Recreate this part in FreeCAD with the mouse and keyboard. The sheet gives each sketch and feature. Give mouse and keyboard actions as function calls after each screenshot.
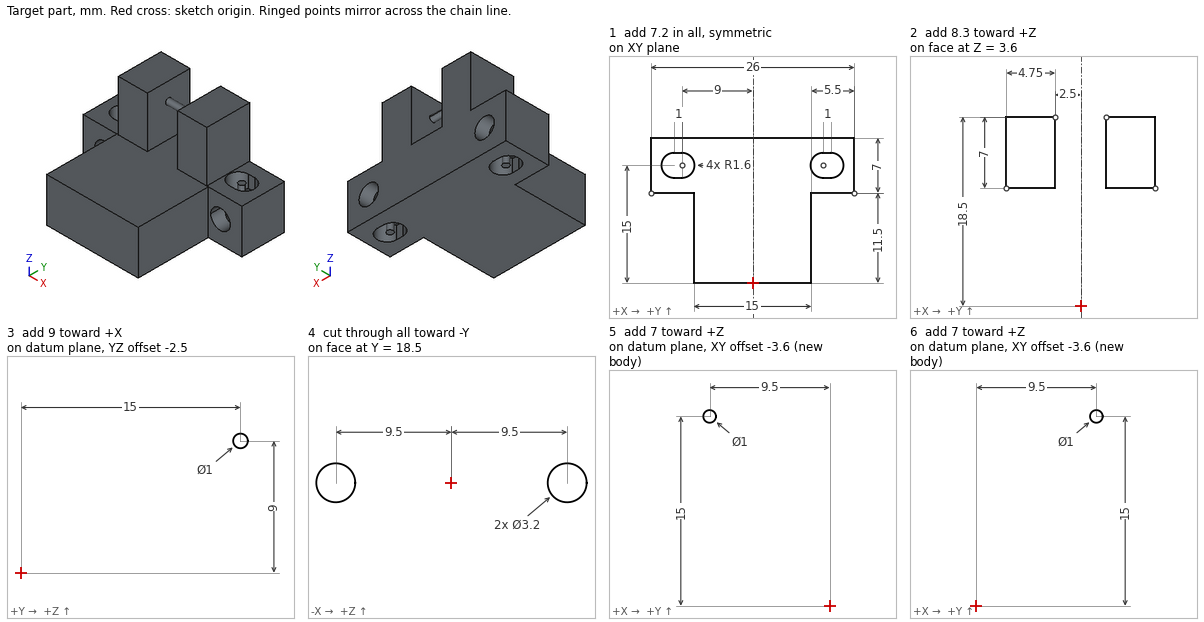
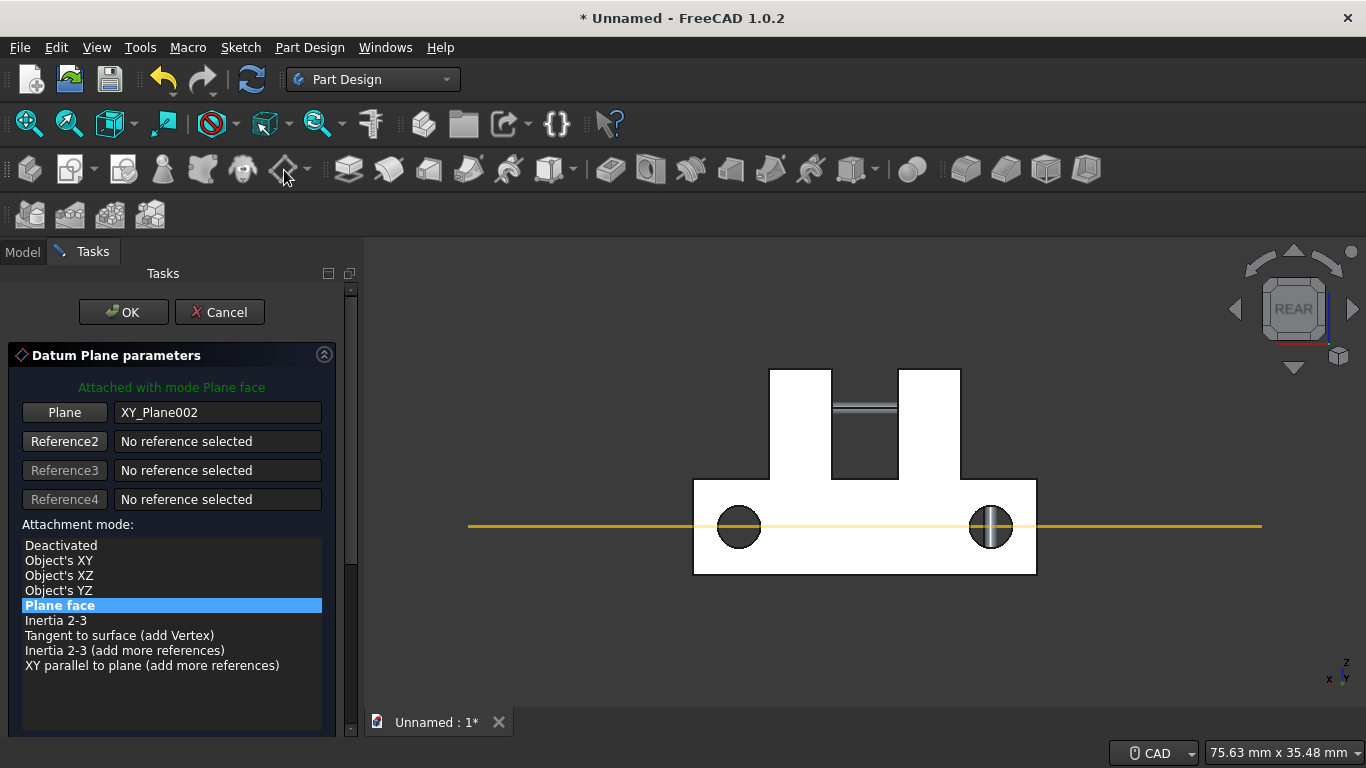
scroll(351, 510, down, 3)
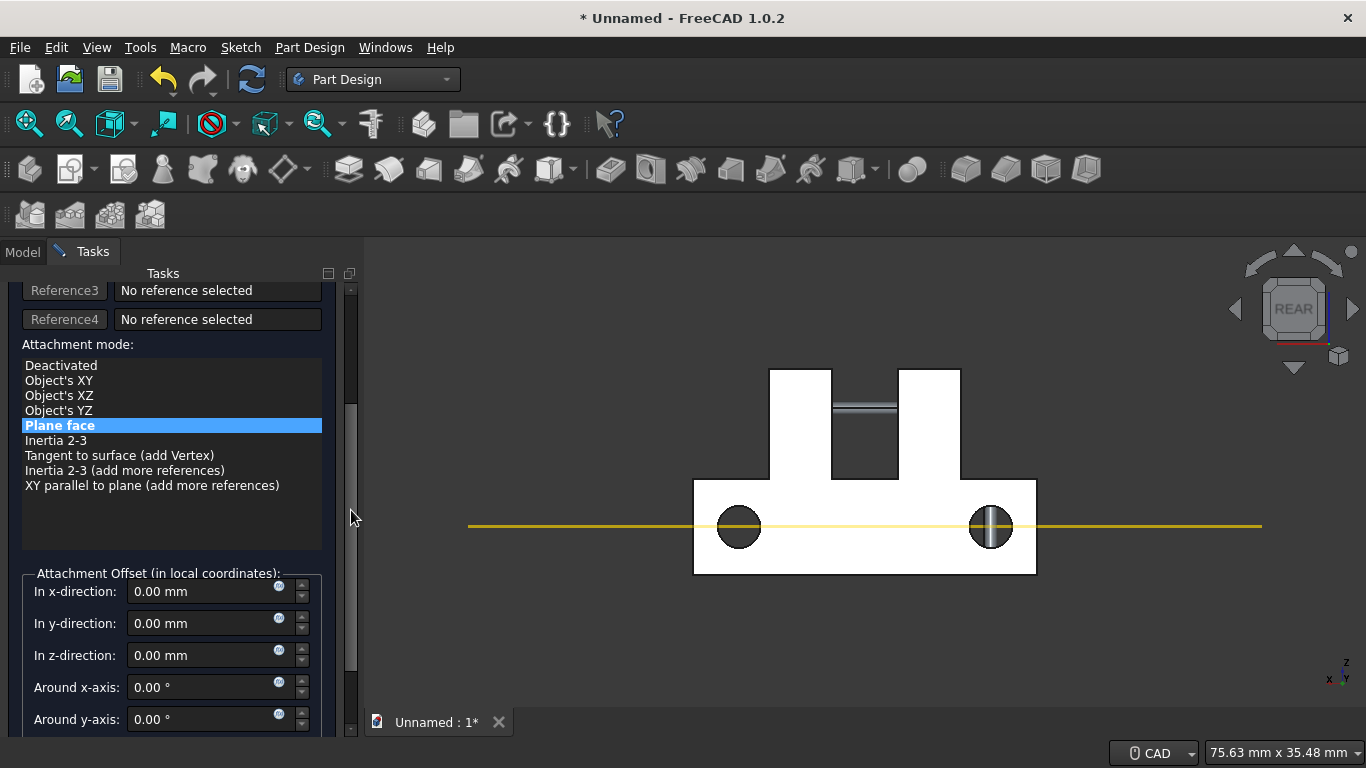
triple_click(210, 655)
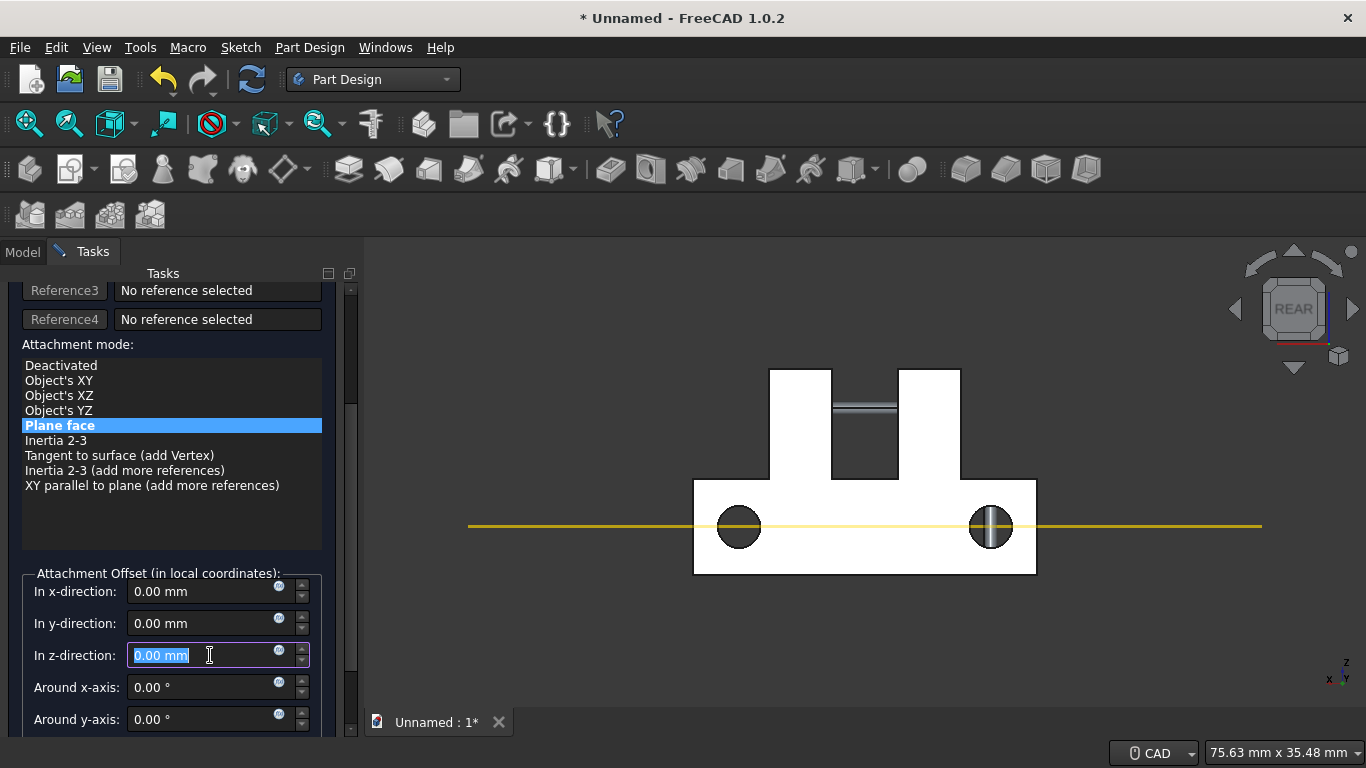
text(-3.6)
key(Tab)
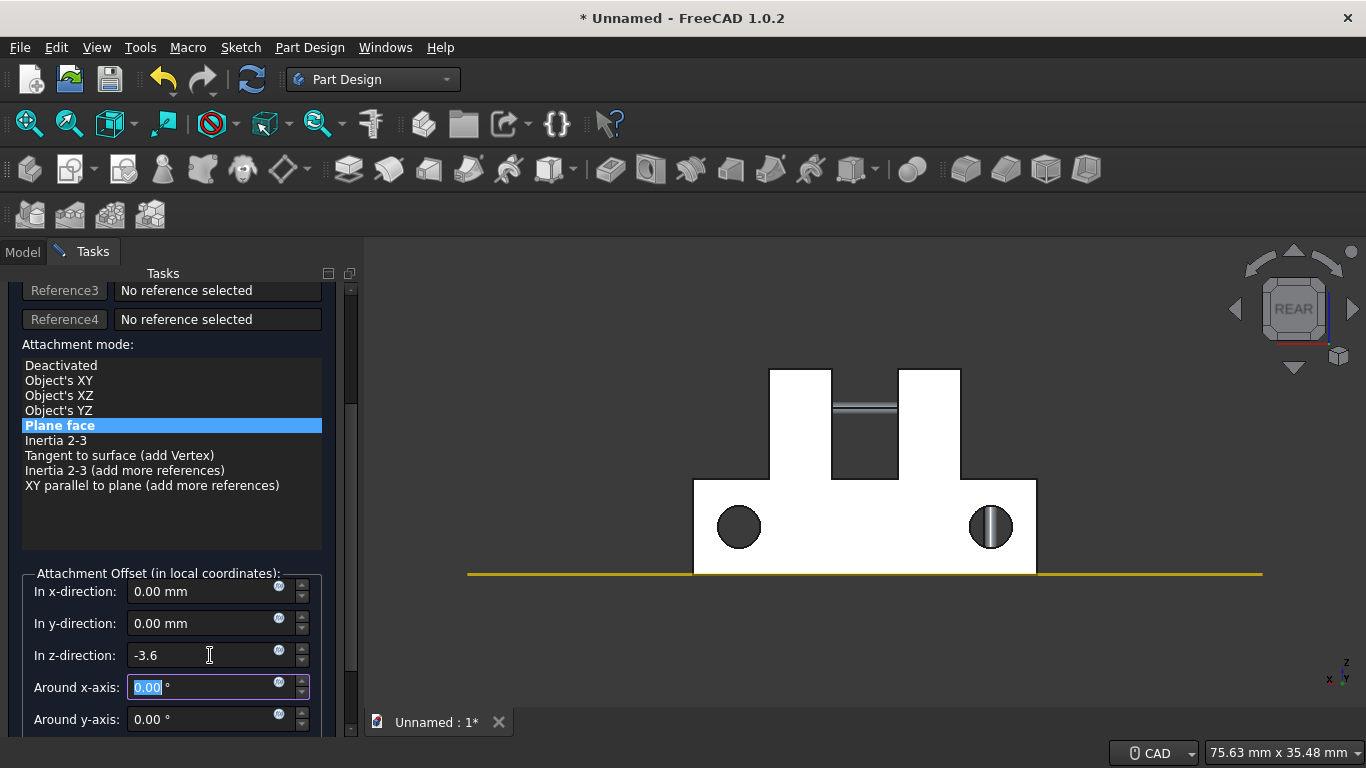
scroll(351, 510, up, 4)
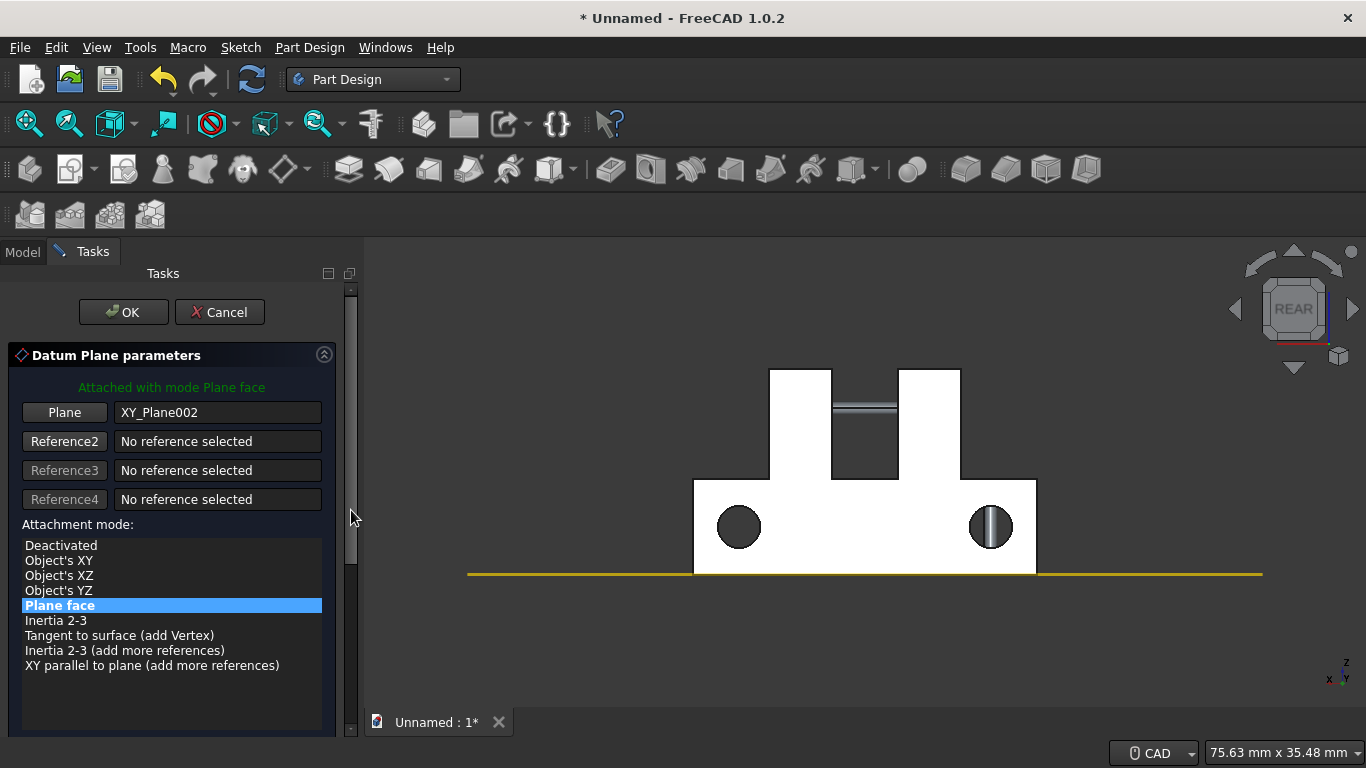
click(124, 312)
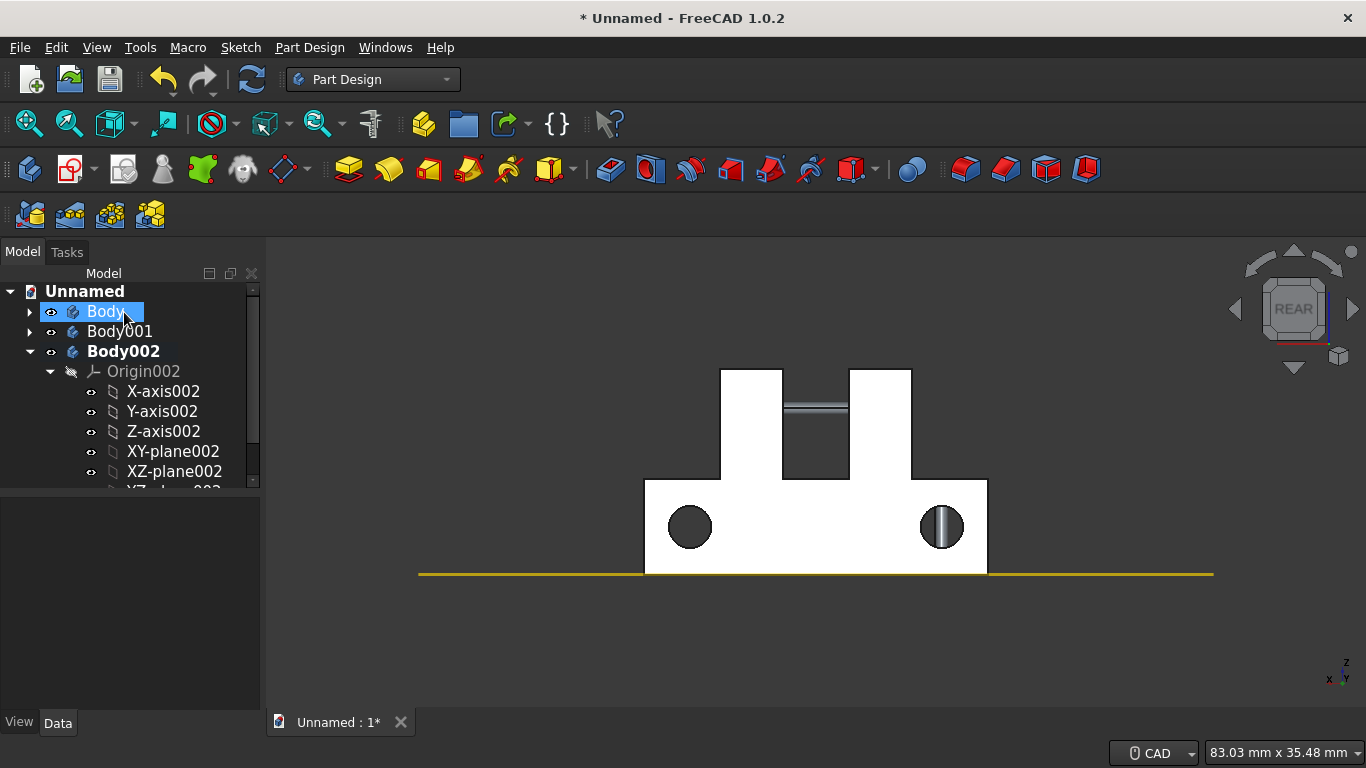
scroll(100, 387, down, 3)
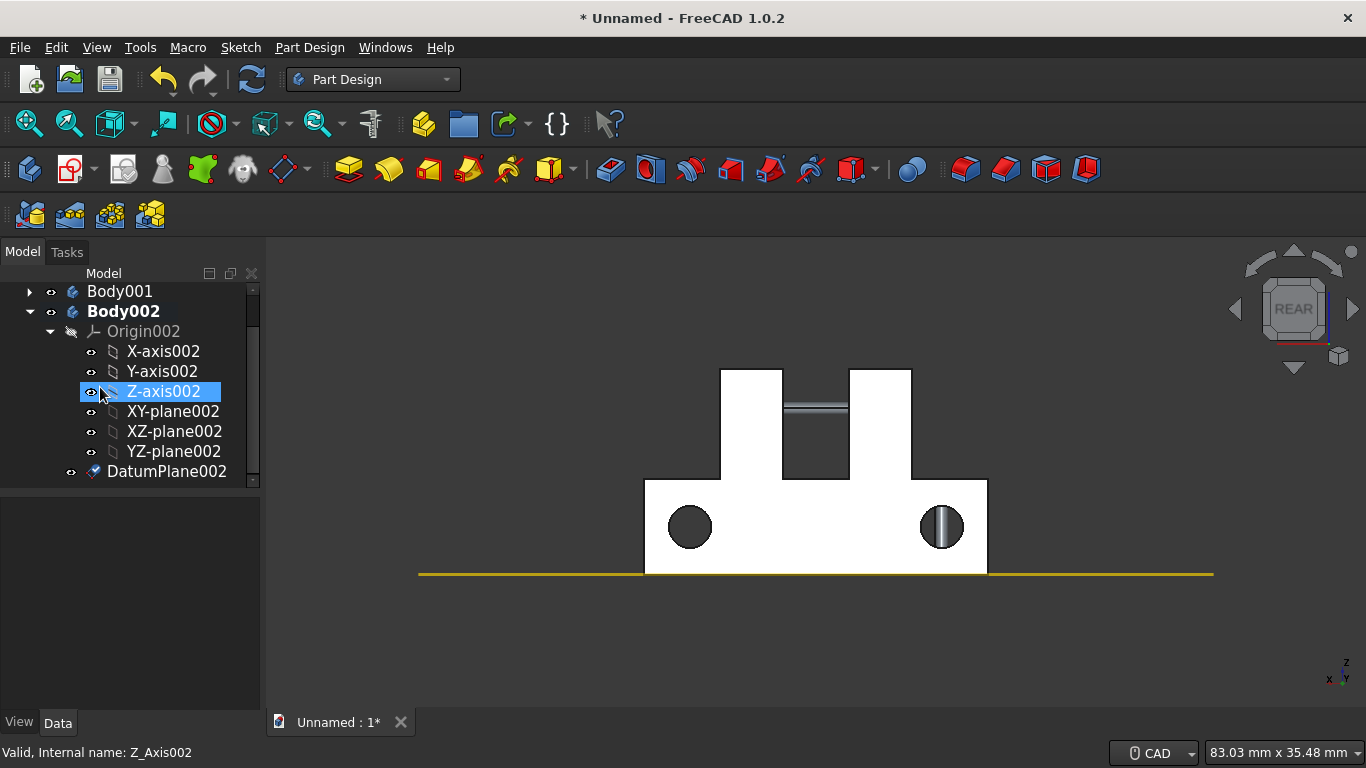
click(116, 472)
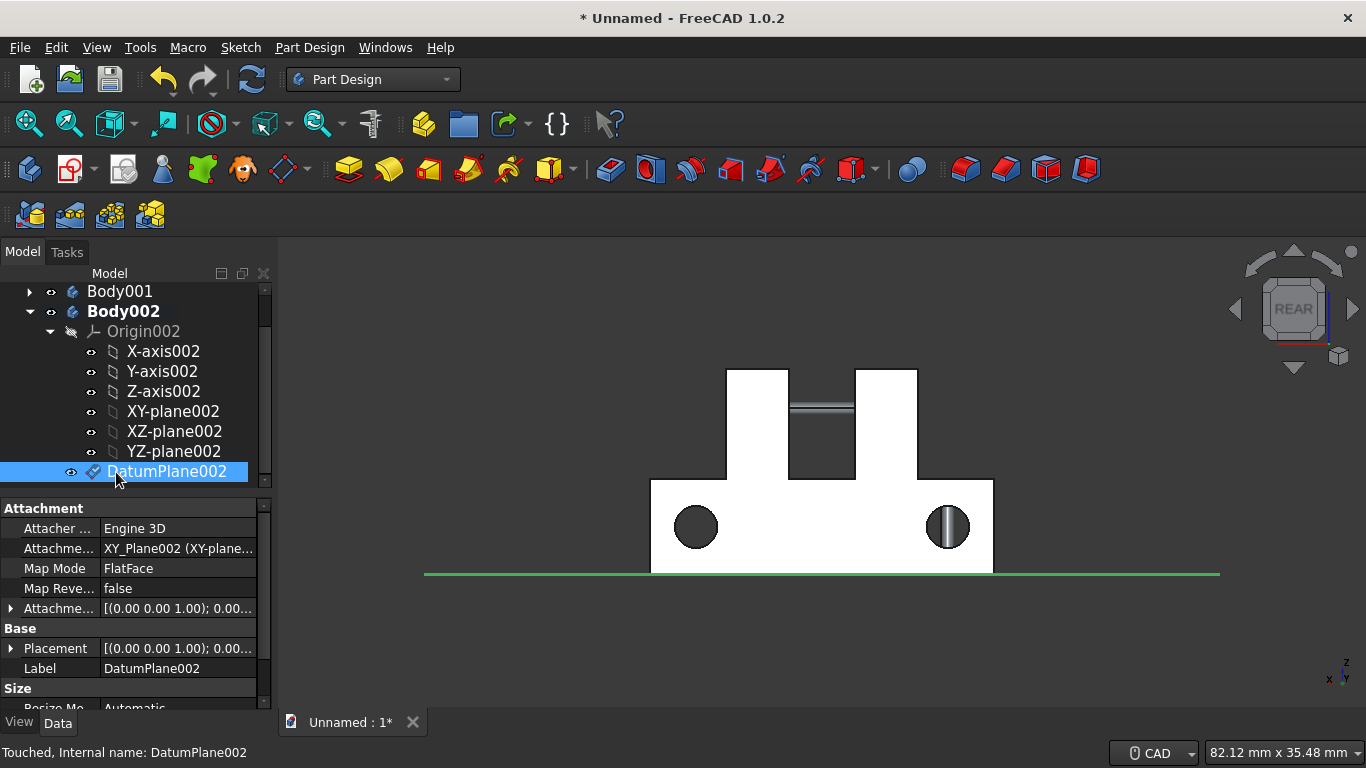
click(70, 170)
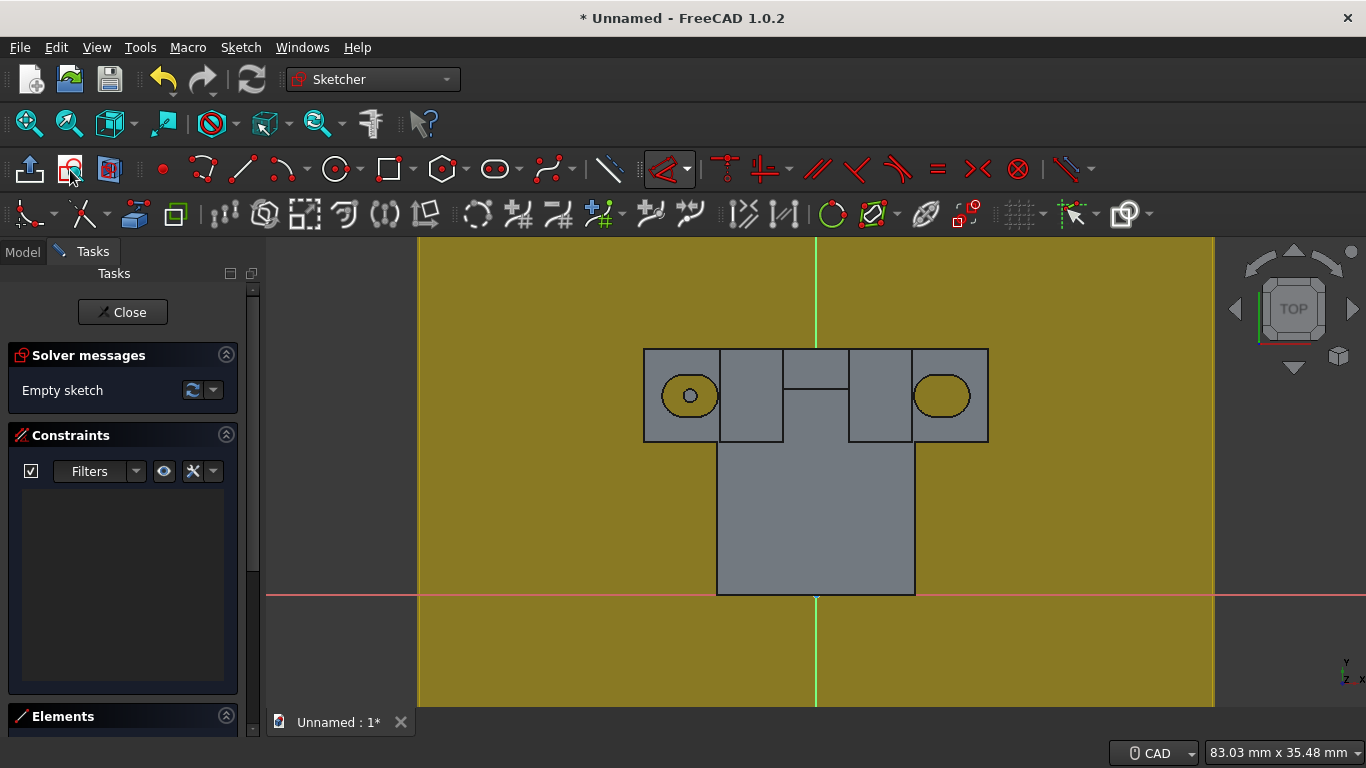
scroll(952, 392, up, 15)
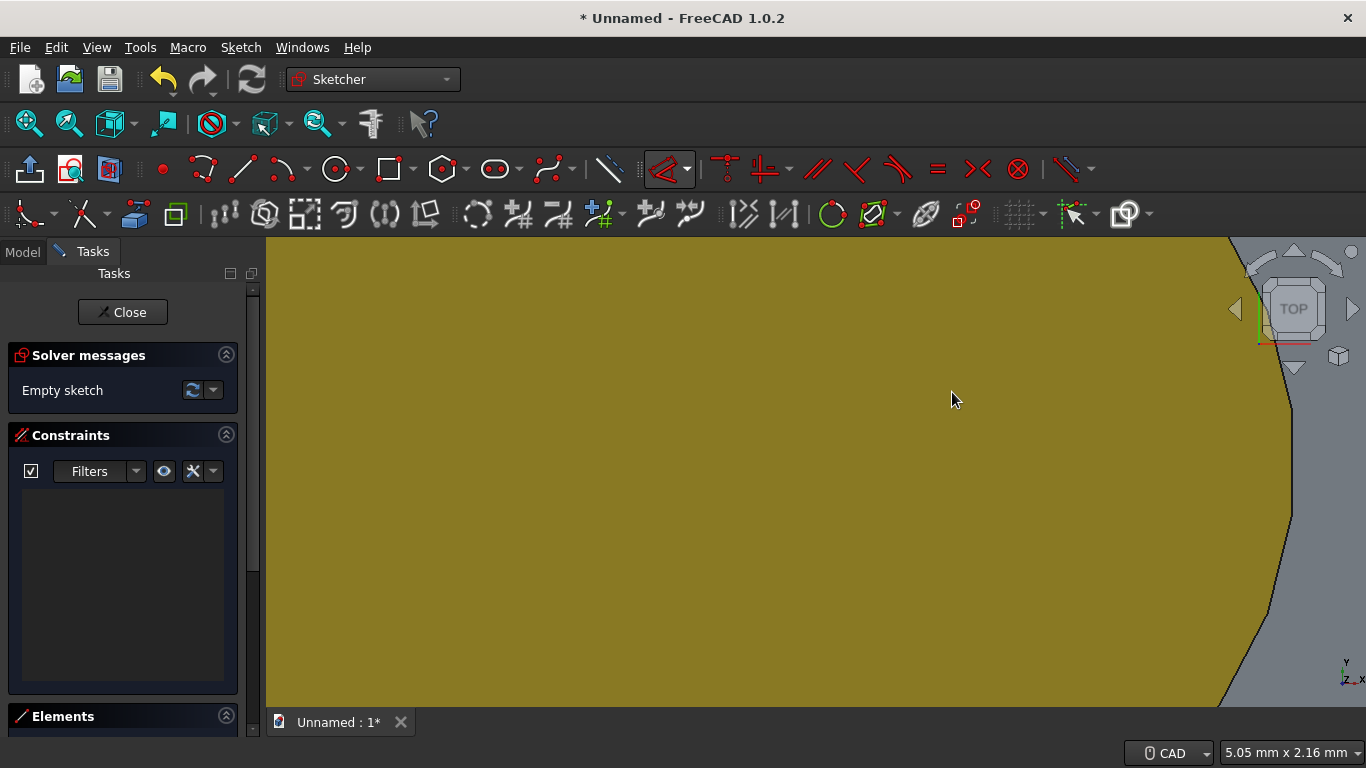
click(336, 170)